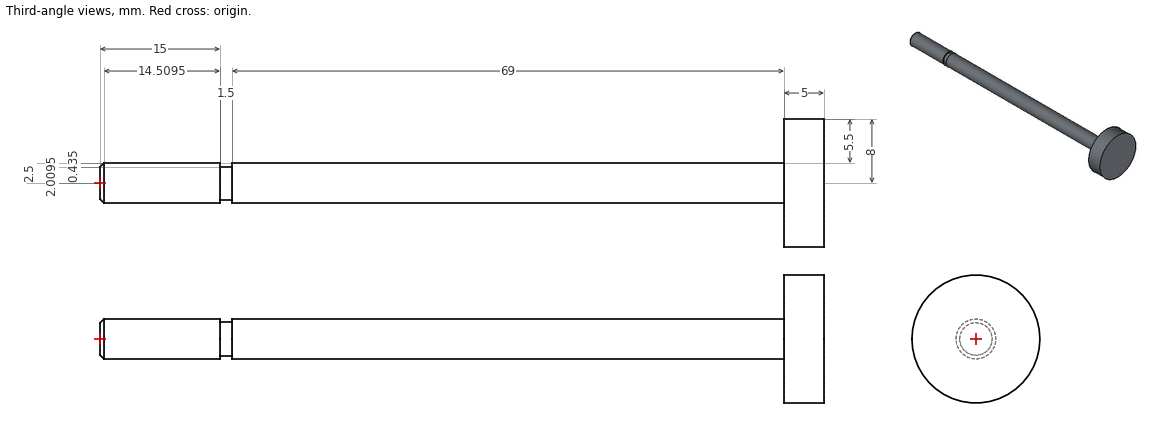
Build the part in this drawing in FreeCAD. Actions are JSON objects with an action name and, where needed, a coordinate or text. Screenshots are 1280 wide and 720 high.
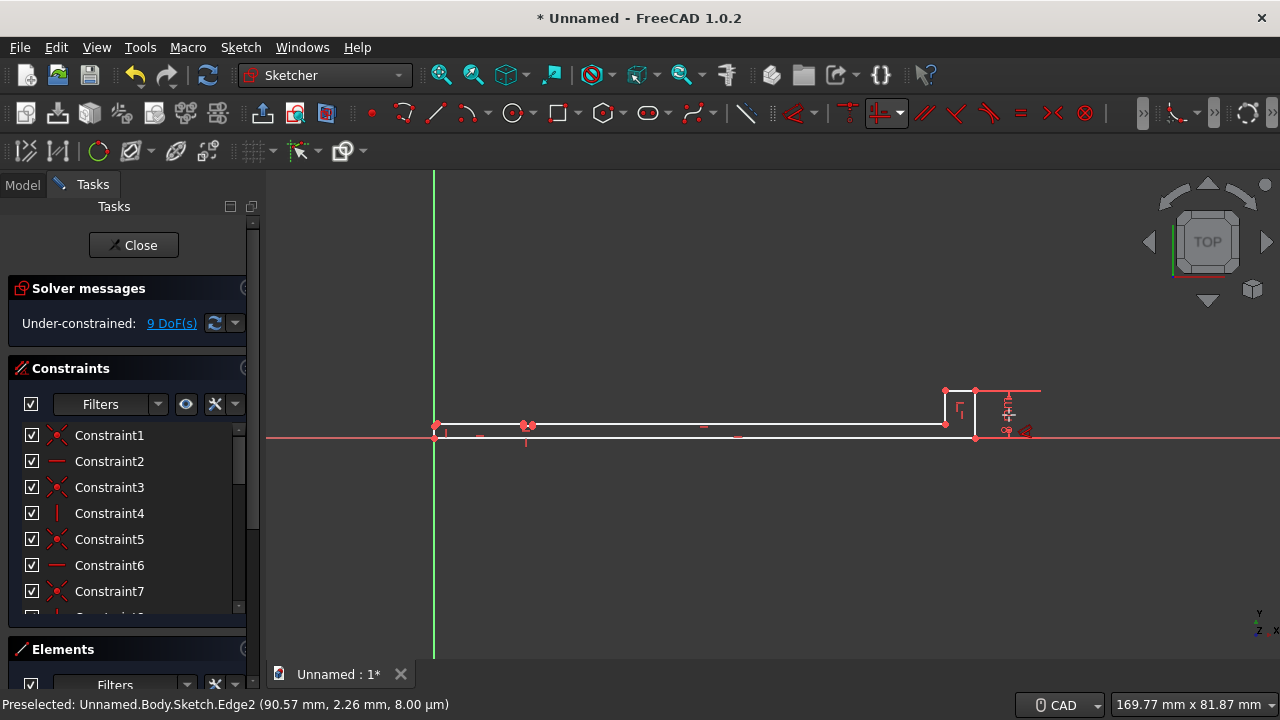
{"action": "scroll", "coordinate": [963, 391], "scroll_direction": "up", "scroll_amount": 2}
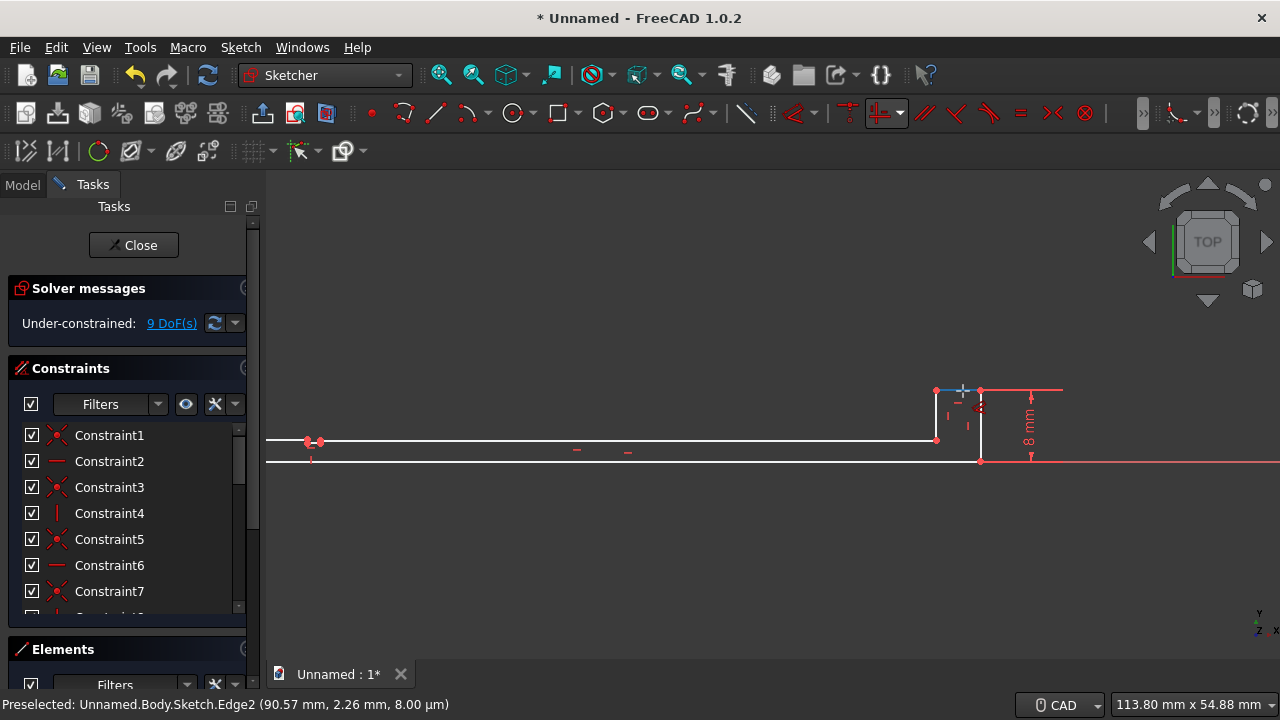
{"action": "left_click", "coordinate": [963, 390]}
{"action": "left_click", "coordinate": [958, 356]}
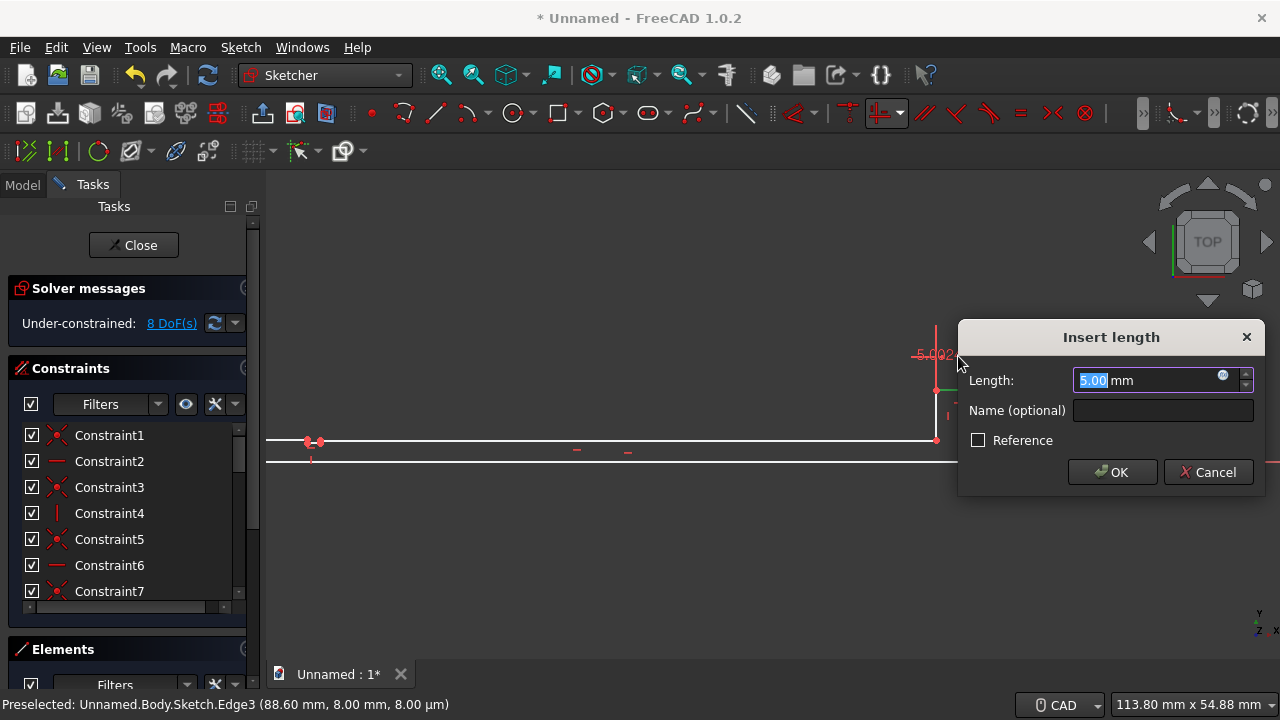
{"action": "type", "text": "5"}
{"action": "key", "text": "Return"}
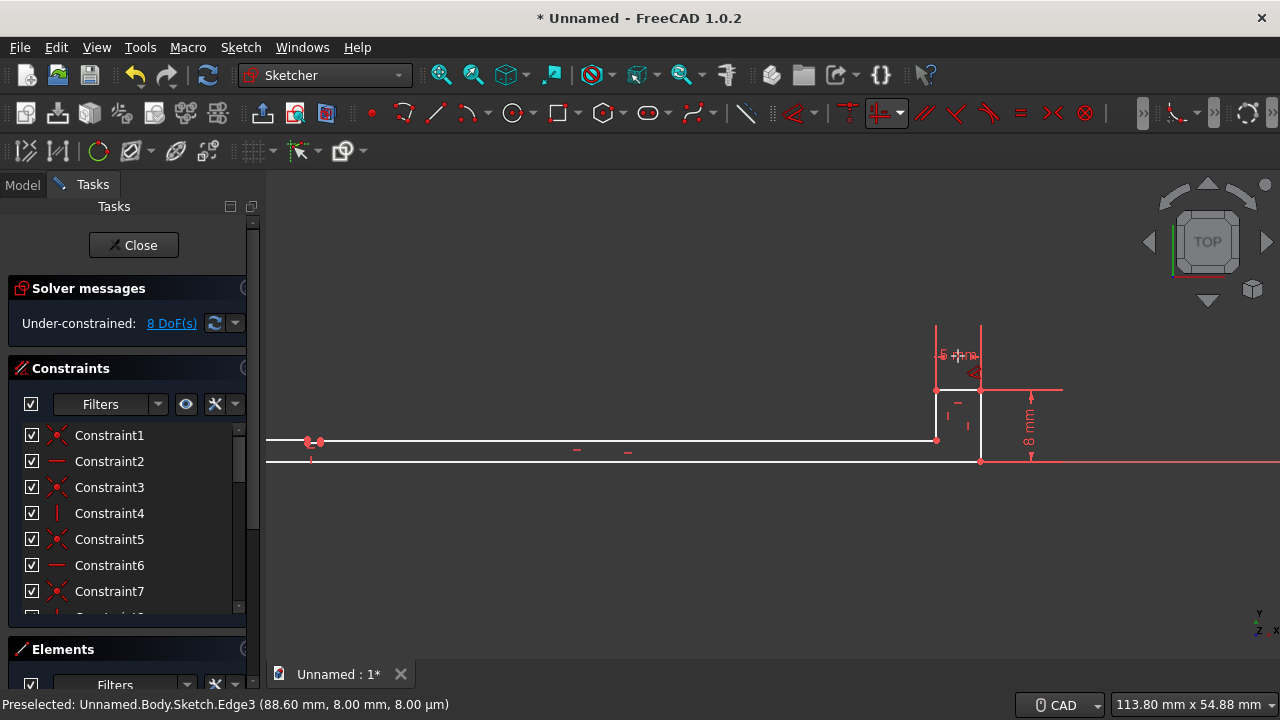
{"action": "left_click", "coordinate": [751, 441]}
{"action": "left_click", "coordinate": [628, 475]}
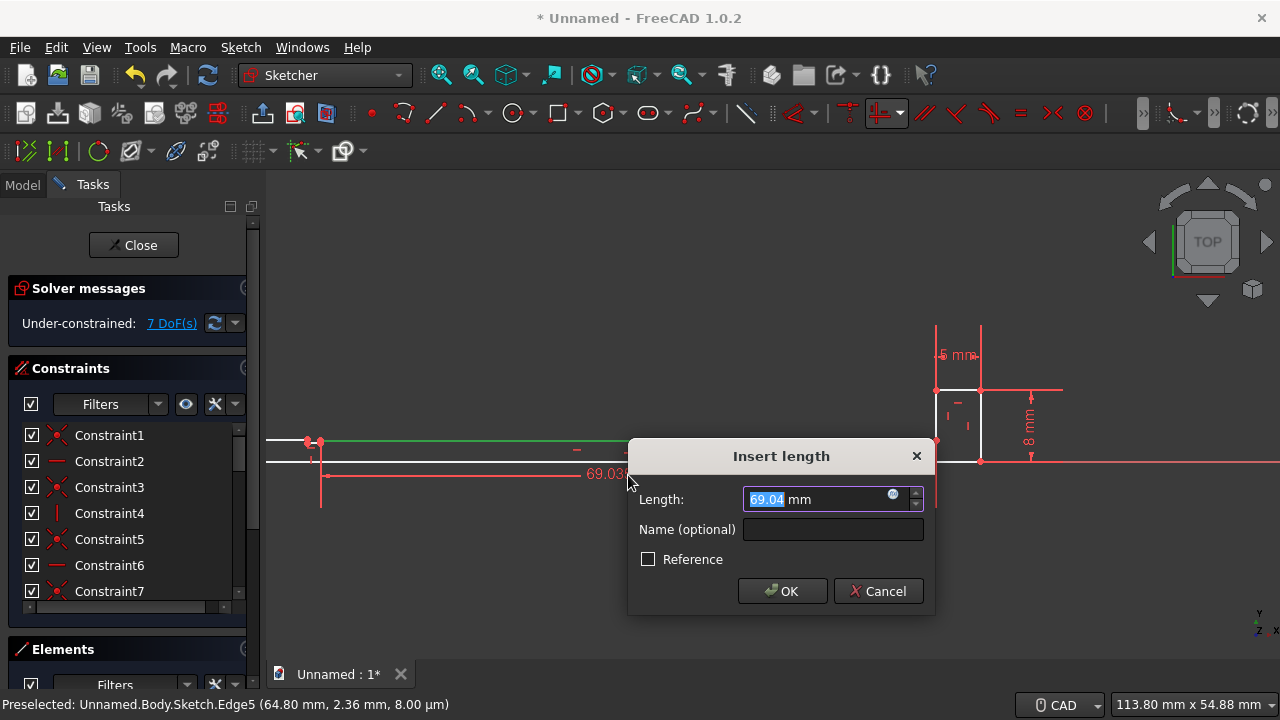
{"action": "type", "text": "69"}
{"action": "key", "text": "Return"}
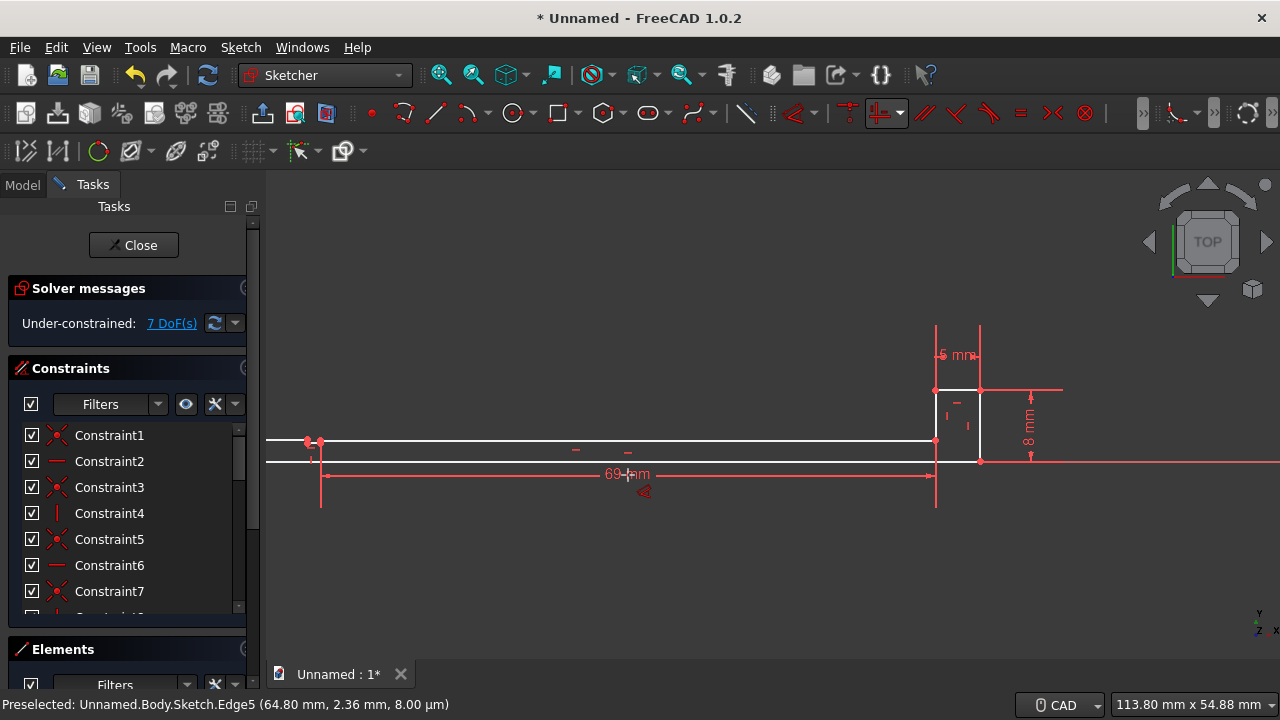
{"action": "left_click", "coordinate": [936, 405]}
{"action": "left_click", "coordinate": [902, 415]}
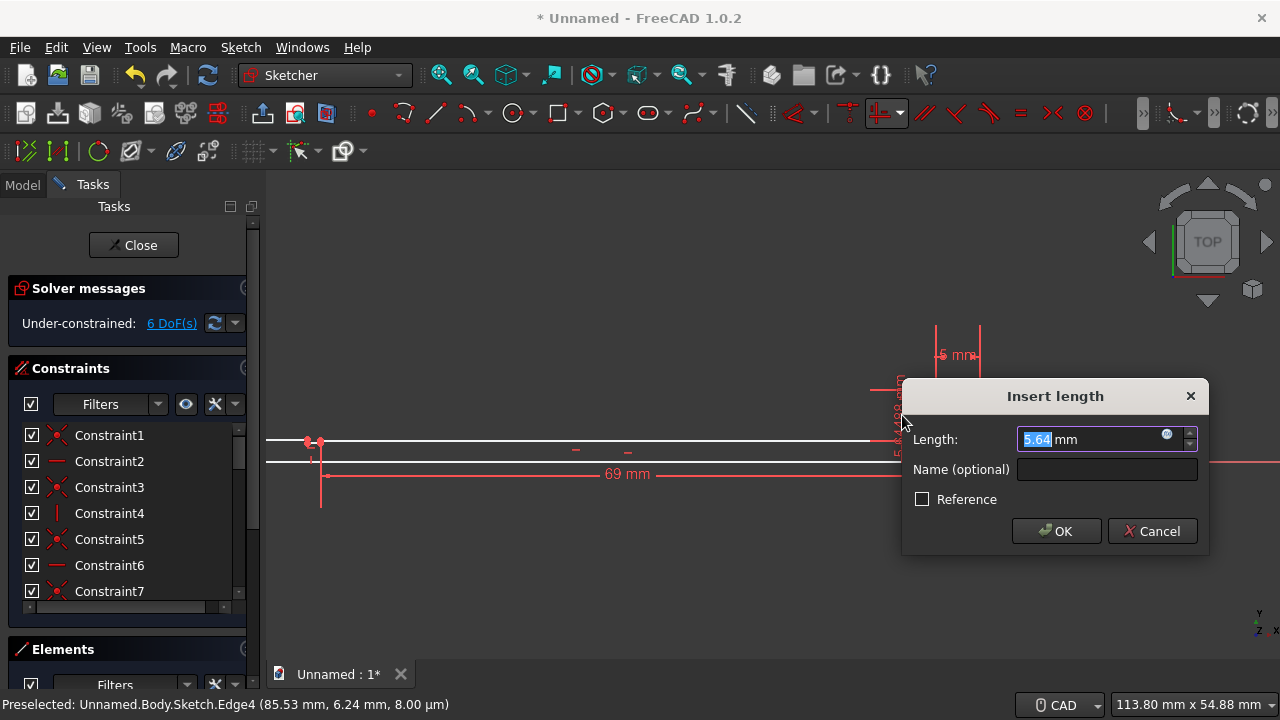
{"action": "type", "text": "5.5"}
{"action": "key", "text": "Return"}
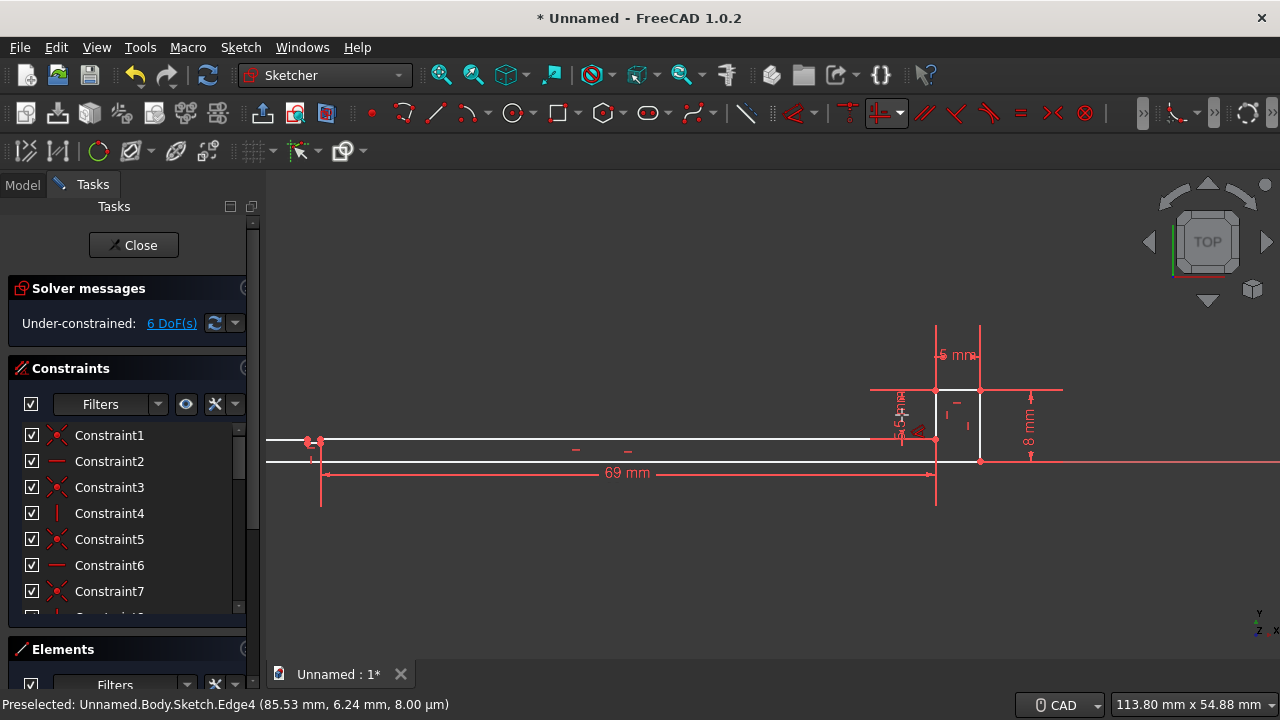
{"action": "scroll", "coordinate": [314, 443], "scroll_direction": "up", "scroll_amount": 6}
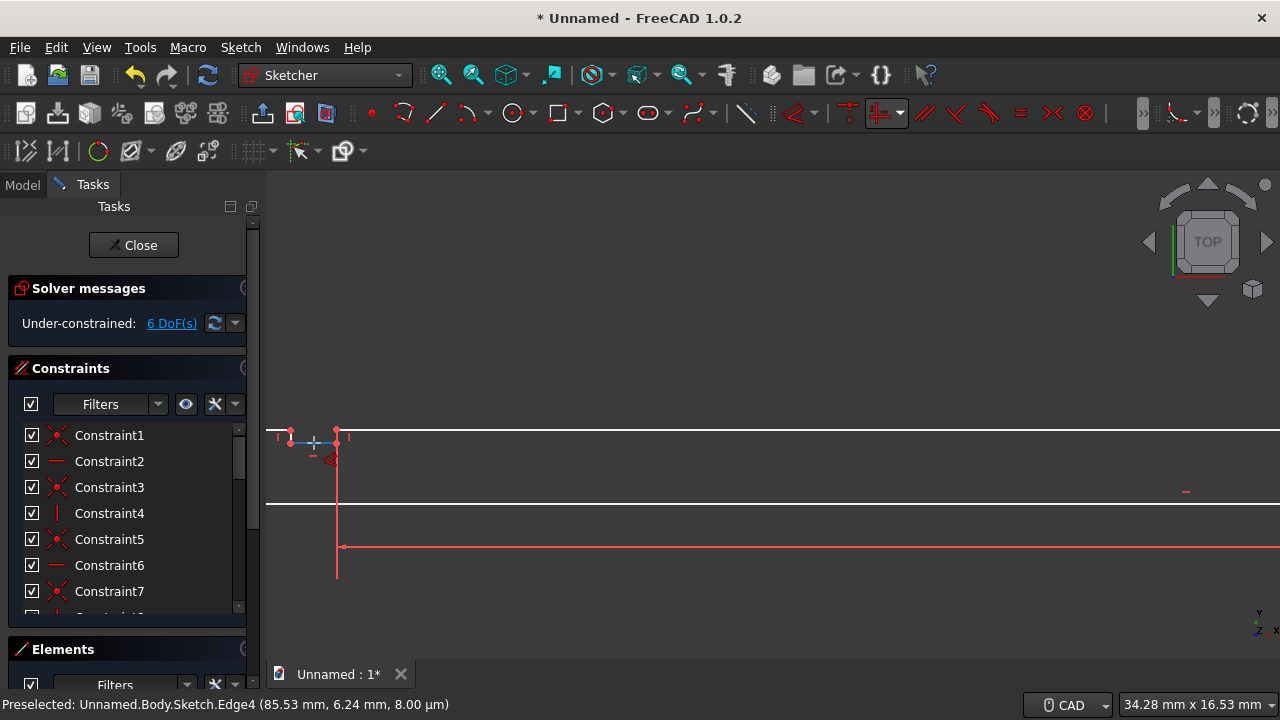
{"action": "left_click", "coordinate": [314, 443]}
{"action": "left_click", "coordinate": [315, 477]}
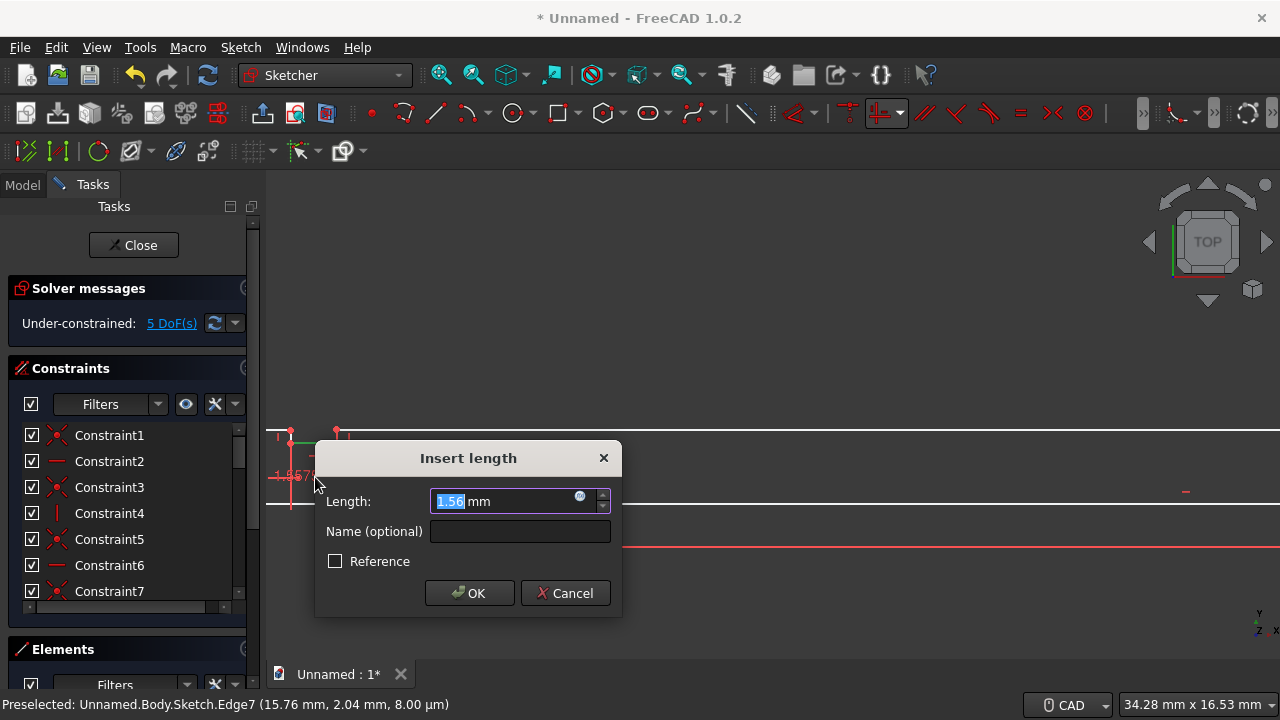
{"action": "type", "text": "1.5"}
{"action": "key", "text": "Return"}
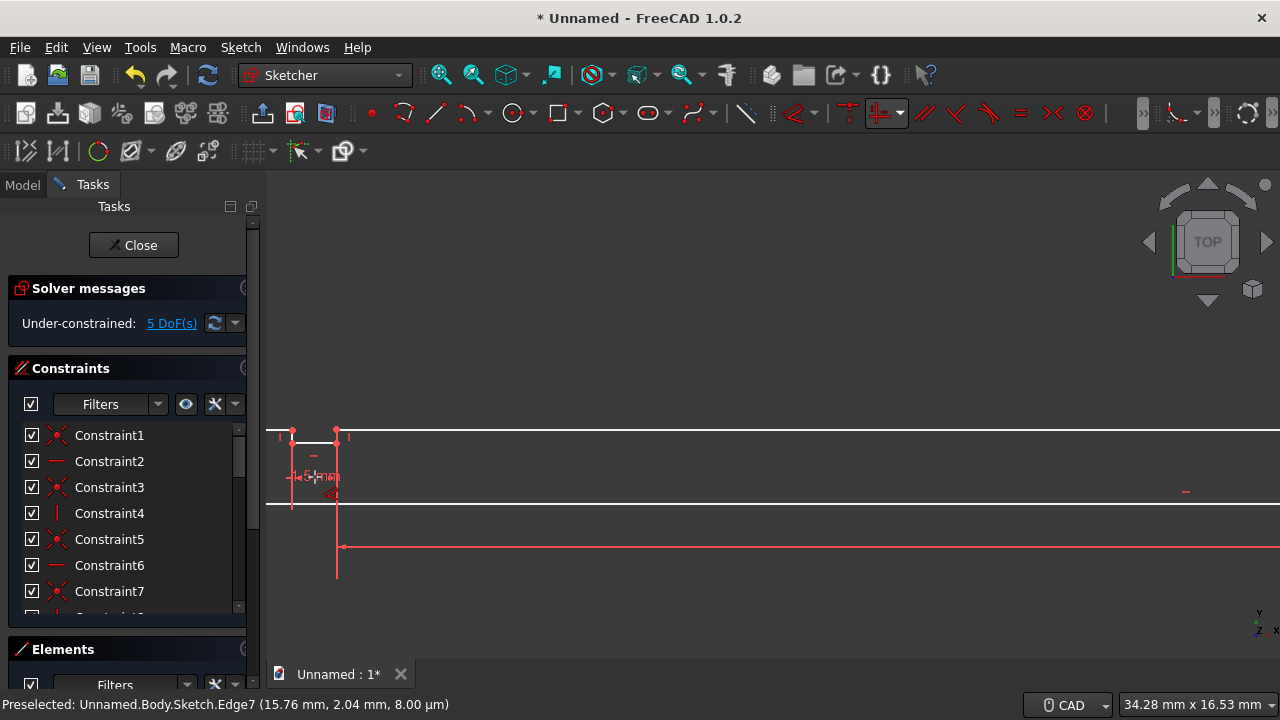
{"action": "scroll", "coordinate": [583, 422], "scroll_direction": "down", "scroll_amount": 8}